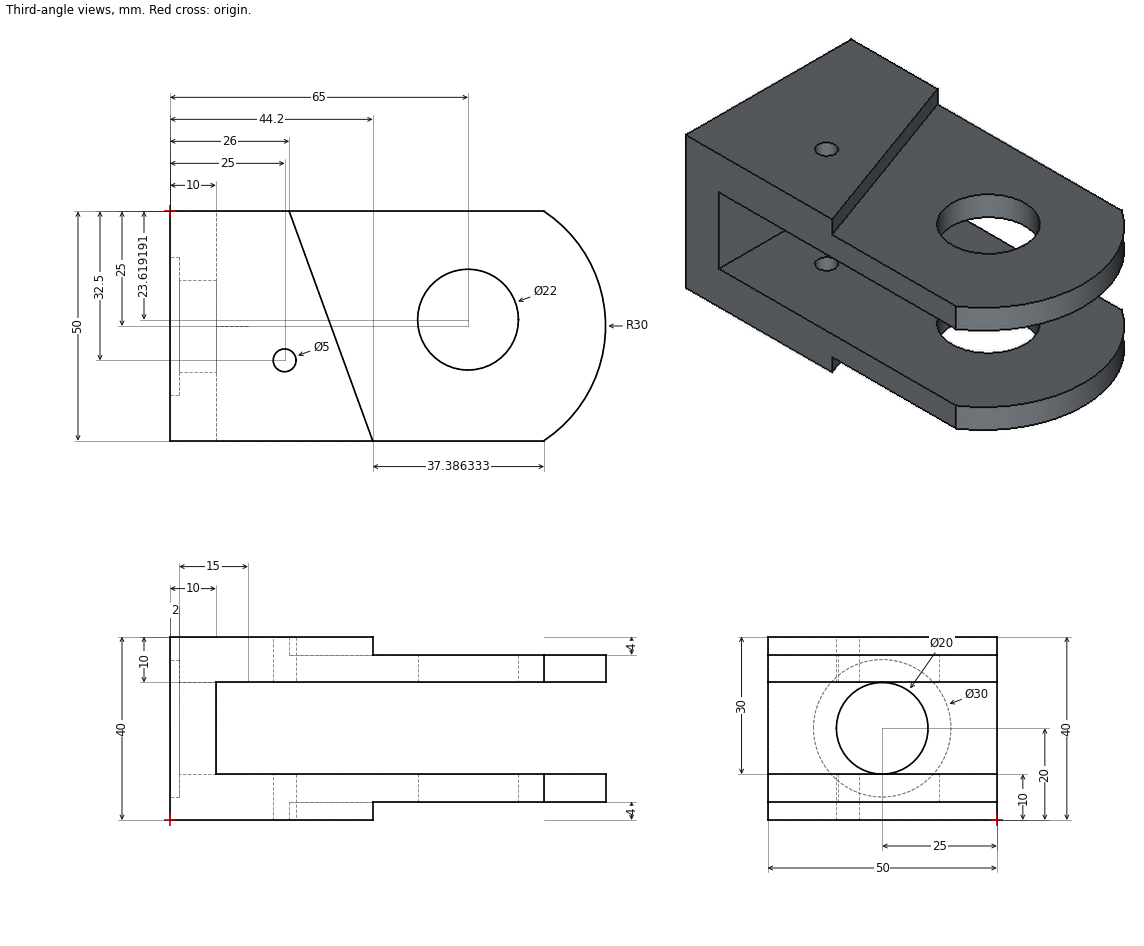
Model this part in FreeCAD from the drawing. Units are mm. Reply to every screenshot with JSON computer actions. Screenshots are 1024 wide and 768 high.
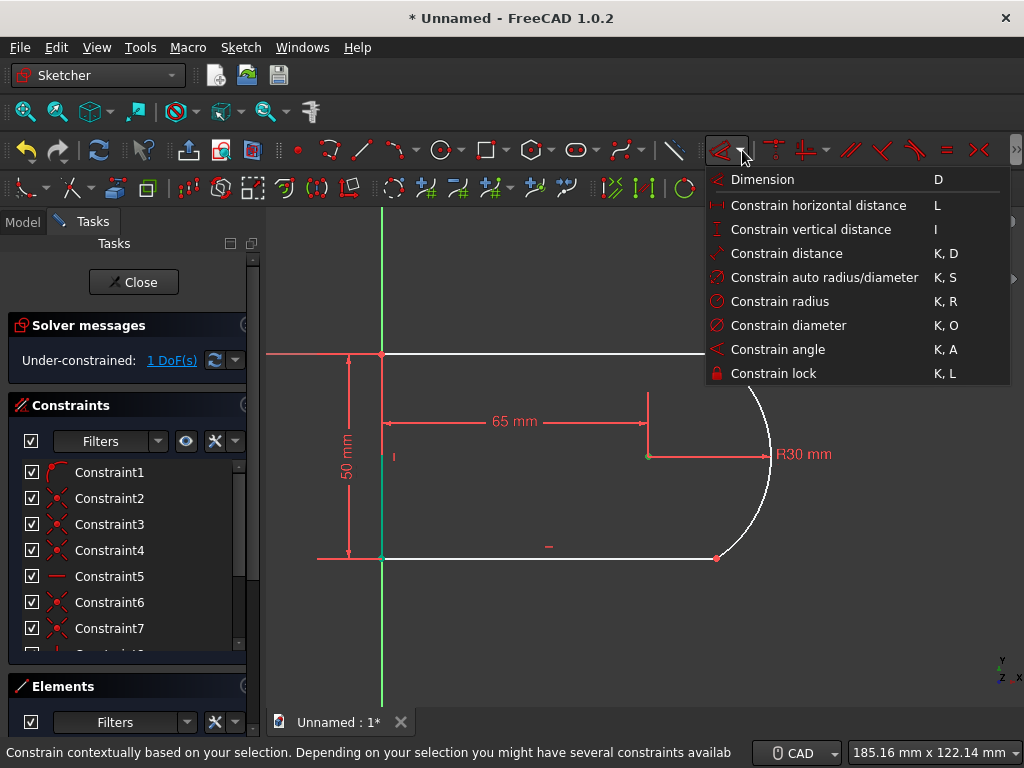
{"action": "left_click", "coordinate": [858, 229]}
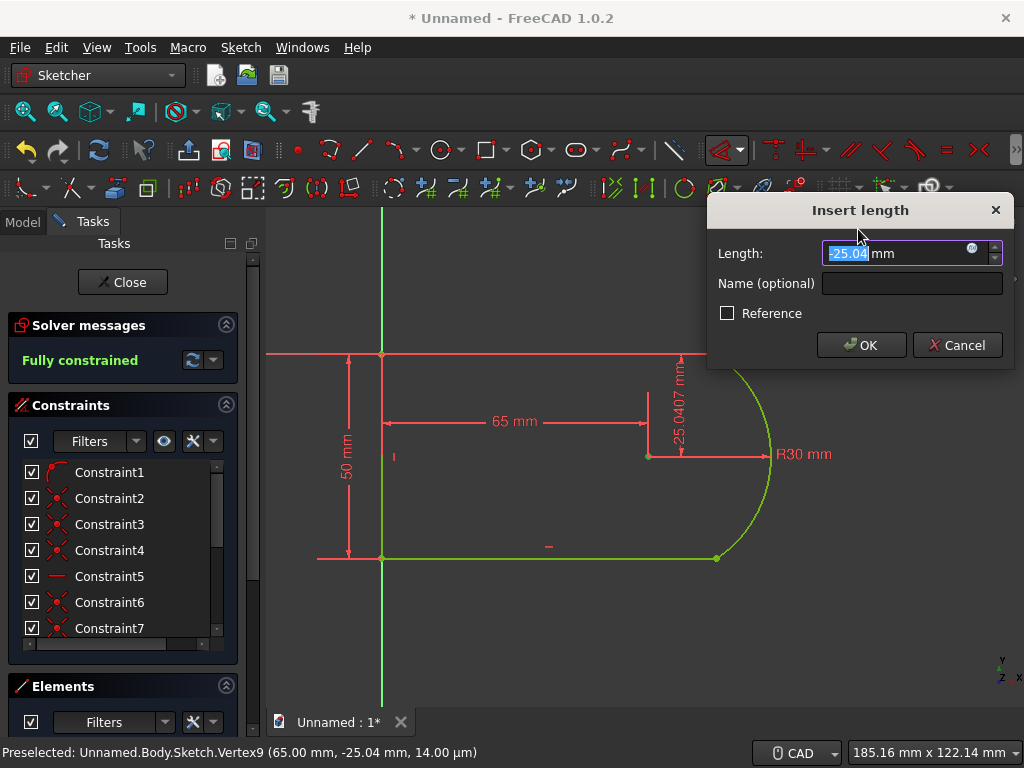
{"action": "type", "text": "-25"}
{"action": "key", "text": "Return"}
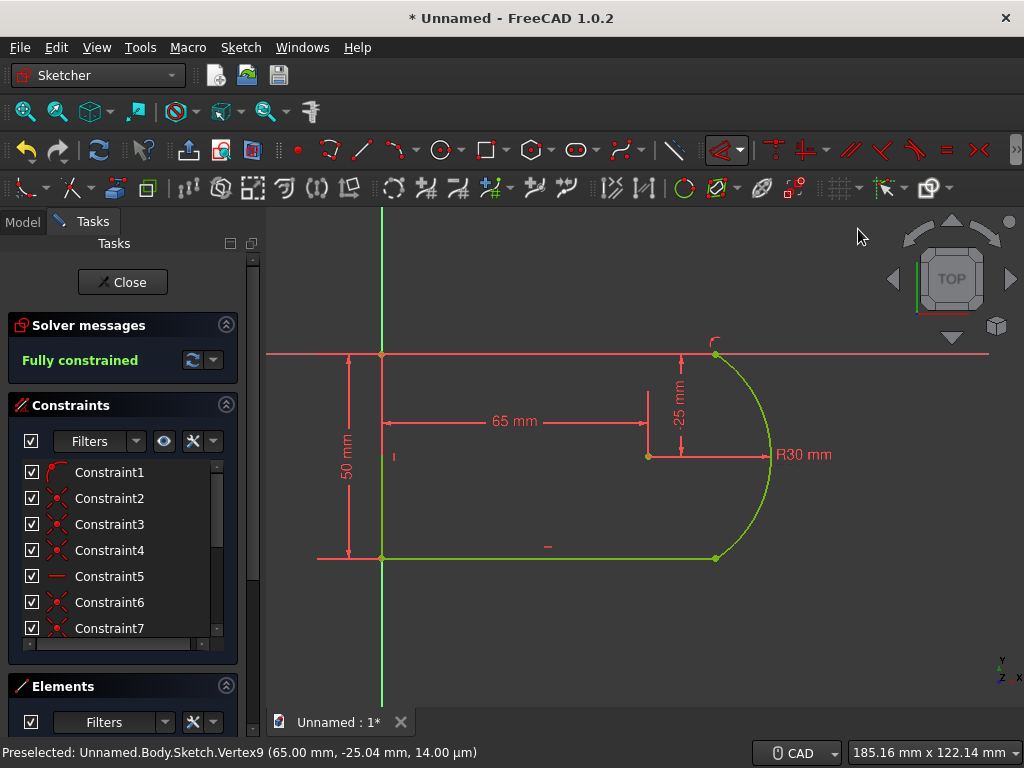
{"action": "left_click", "coordinate": [123, 282]}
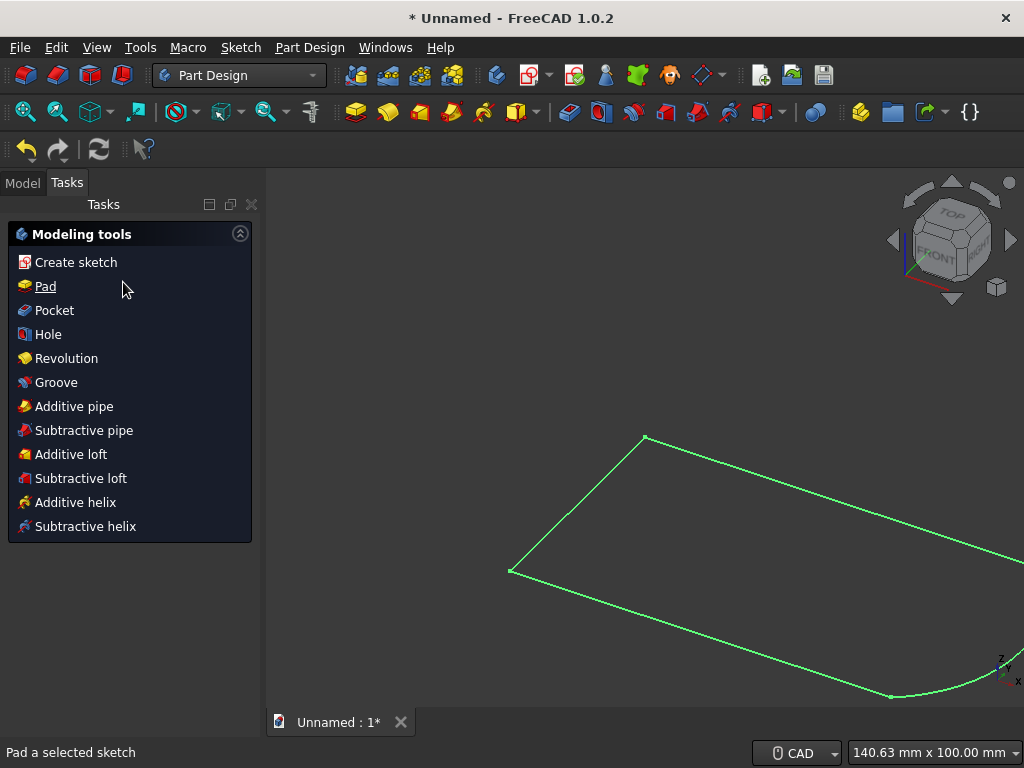
{"action": "left_click", "coordinate": [356, 112]}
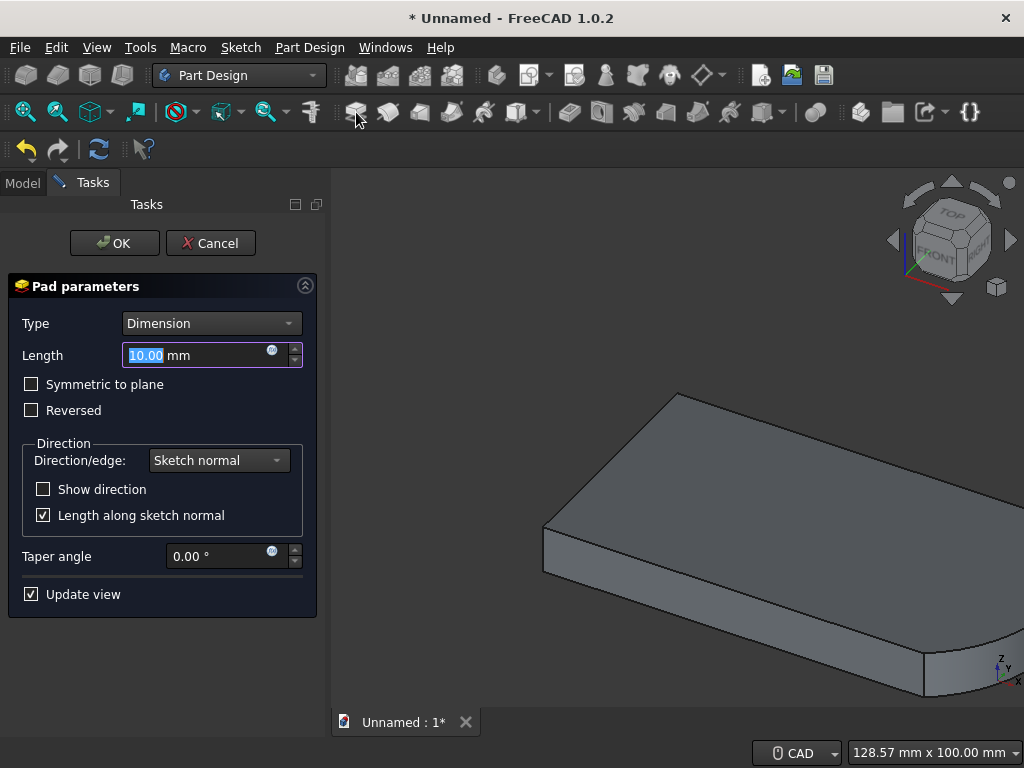
{"action": "type", "text": "10"}
{"action": "key", "text": "Tab"}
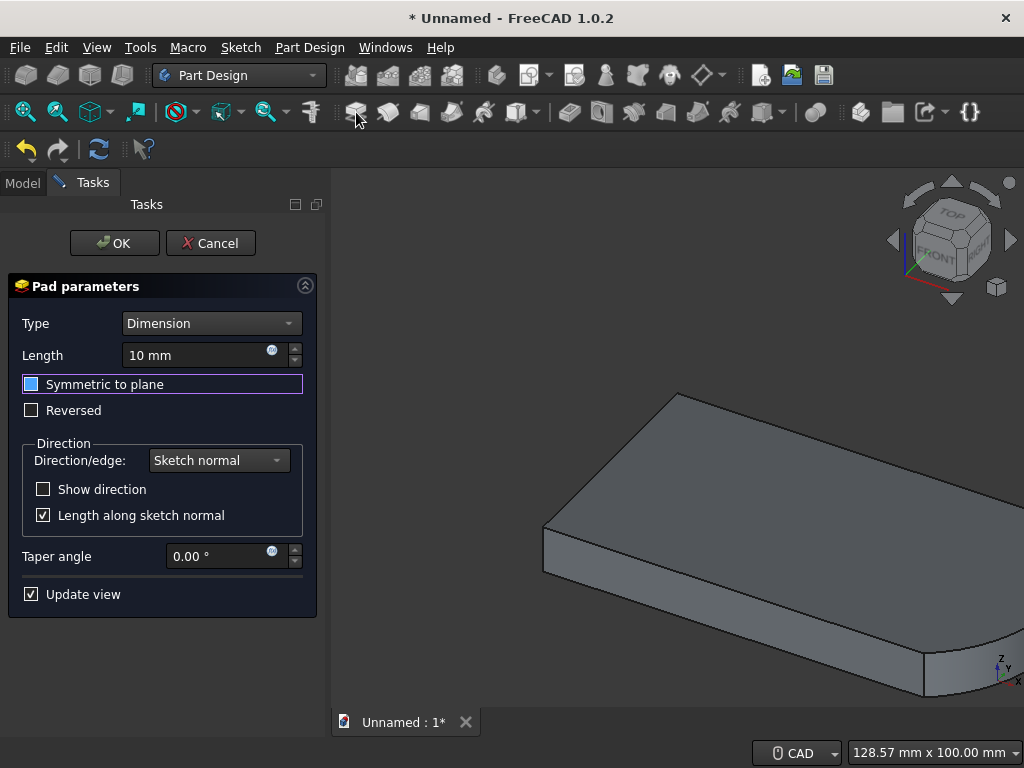
{"action": "left_click", "coordinate": [115, 243]}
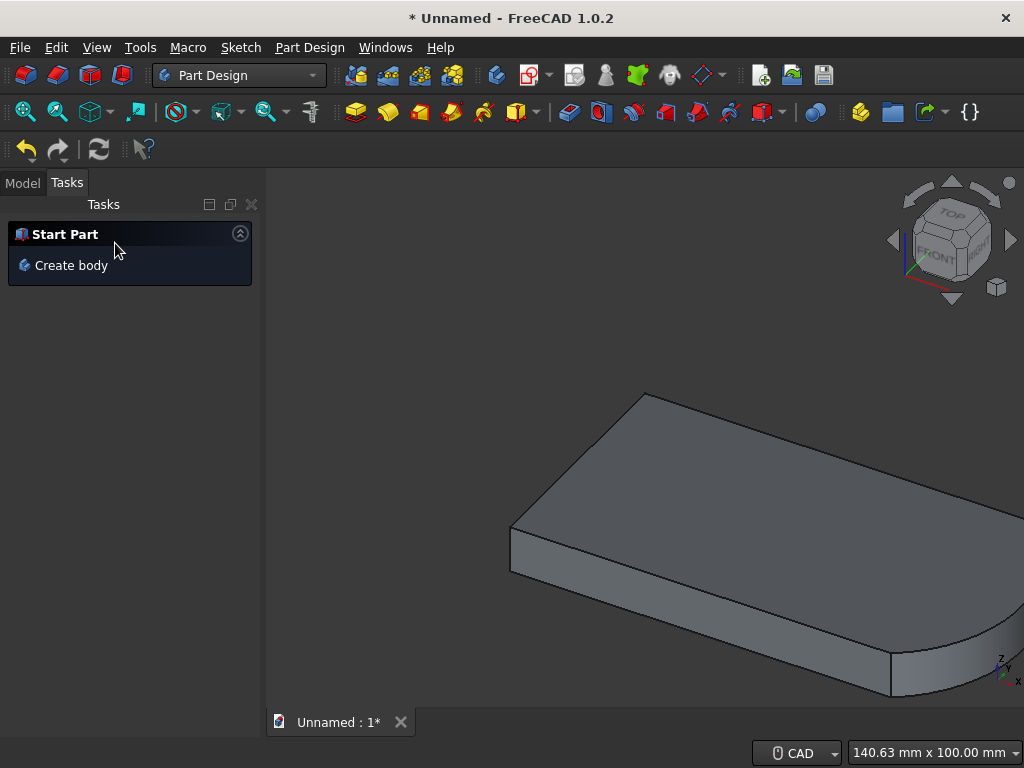
{"action": "left_click", "coordinate": [26, 112]}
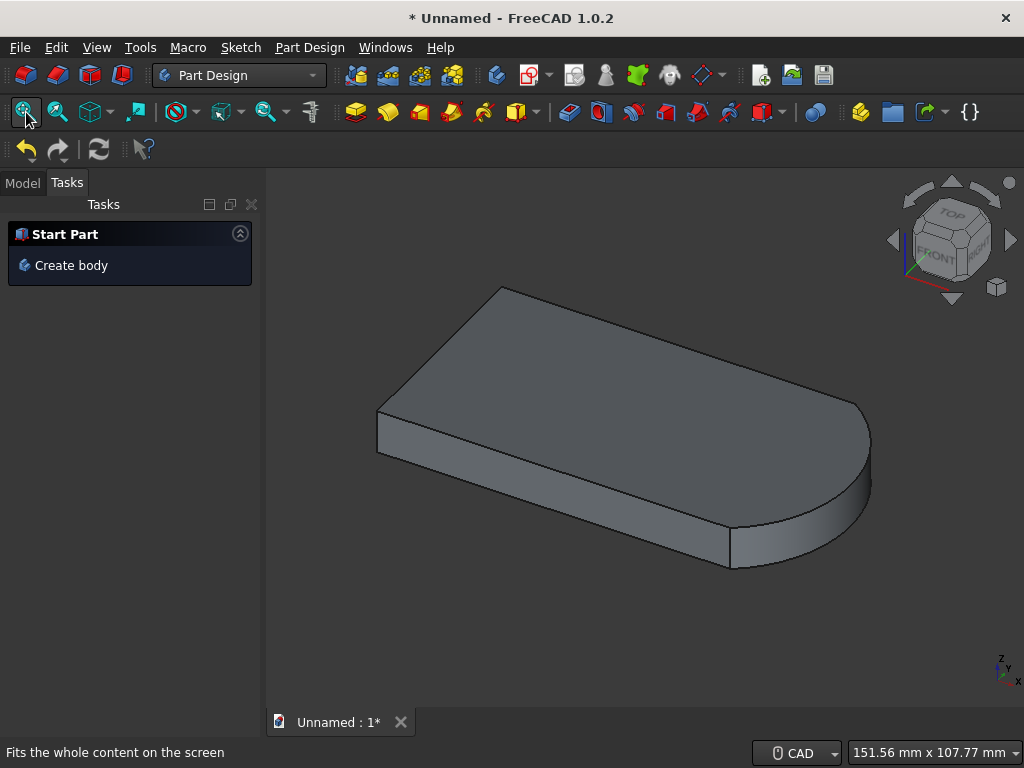
{"action": "left_click", "coordinate": [530, 76]}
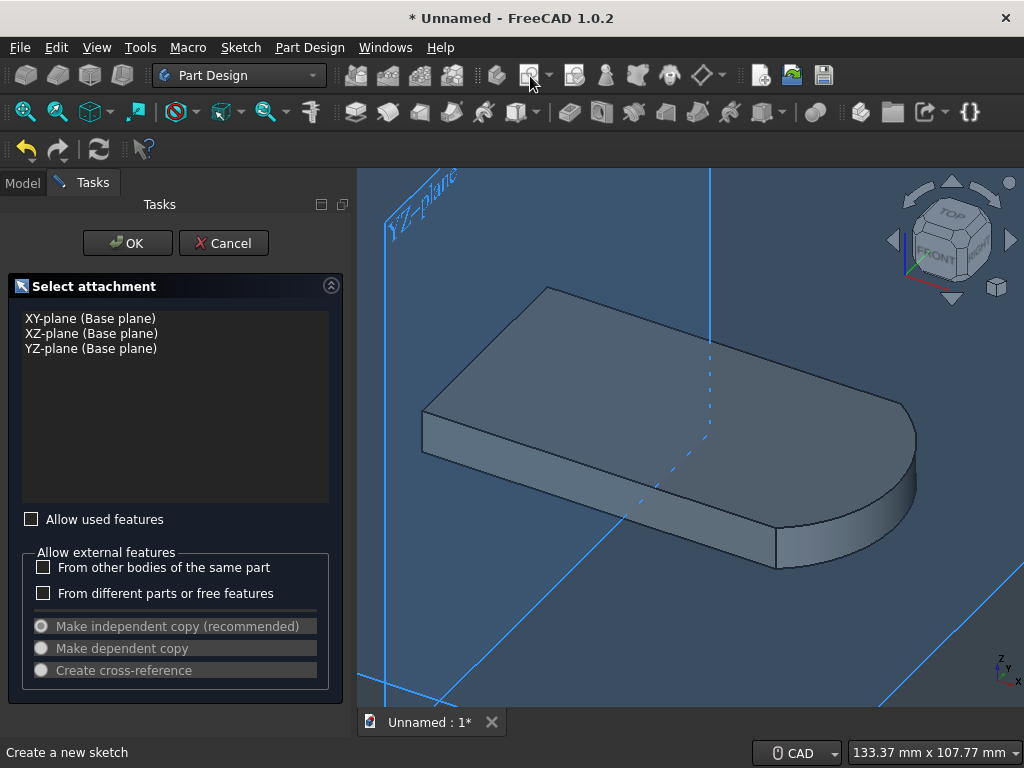
{"action": "left_click", "coordinate": [82, 348]}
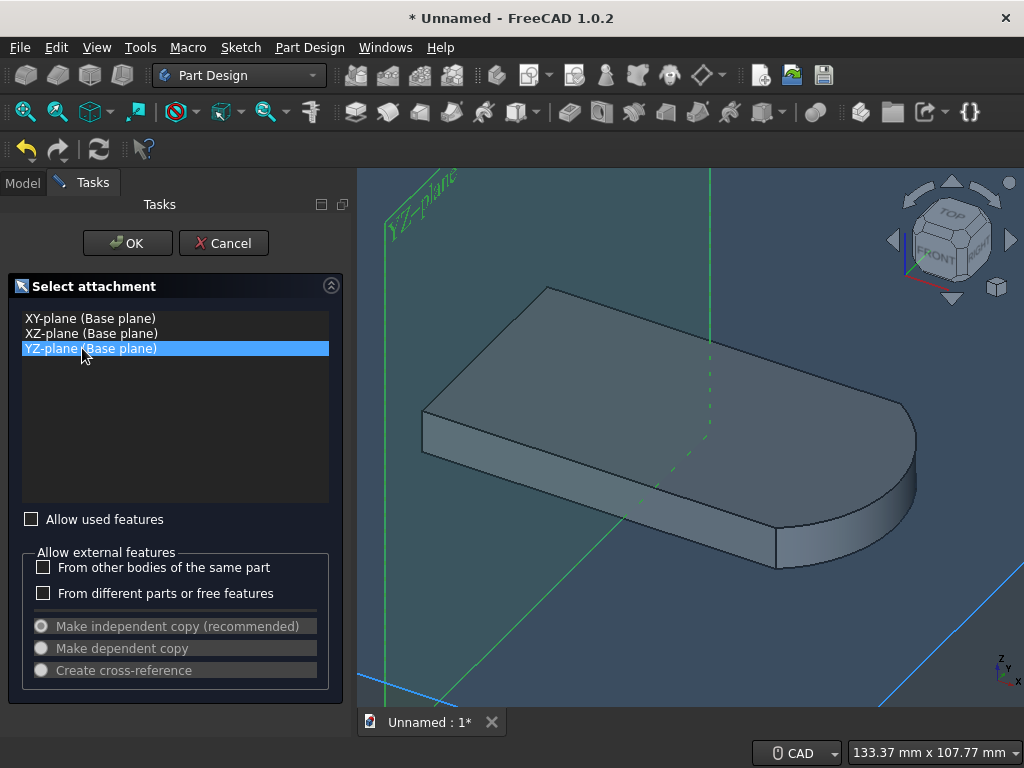
{"action": "left_click", "coordinate": [128, 243]}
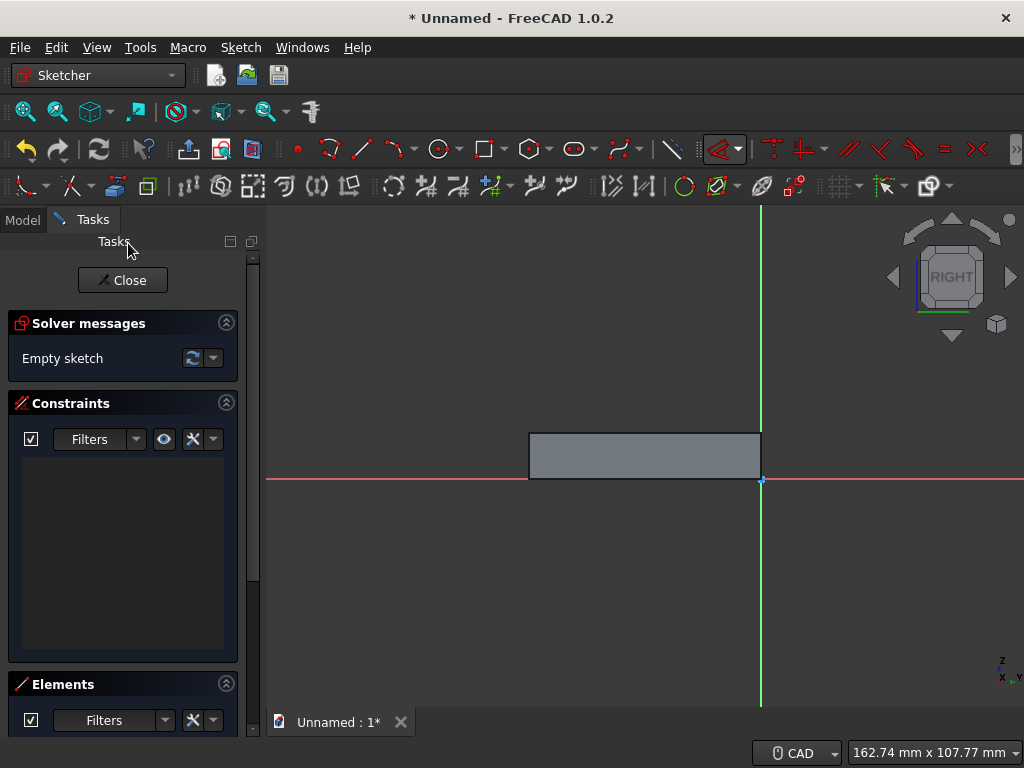
{"action": "left_click", "coordinate": [254, 150]}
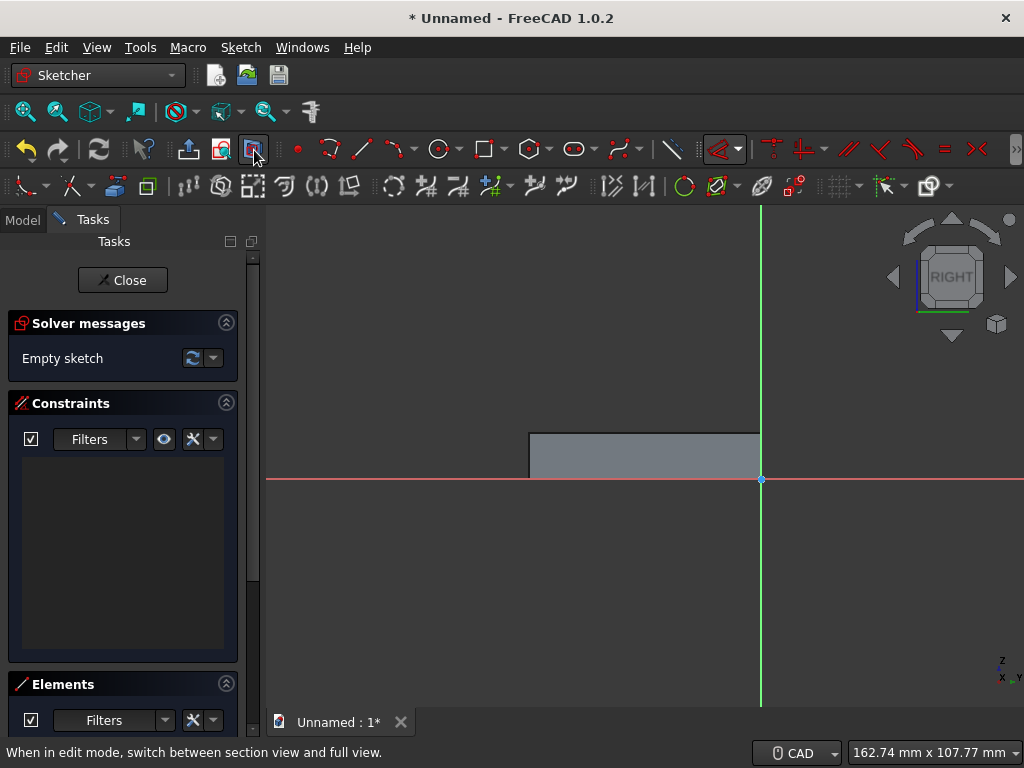
{"action": "scroll", "coordinate": [728, 301], "scroll_direction": "up", "scroll_amount": 3}